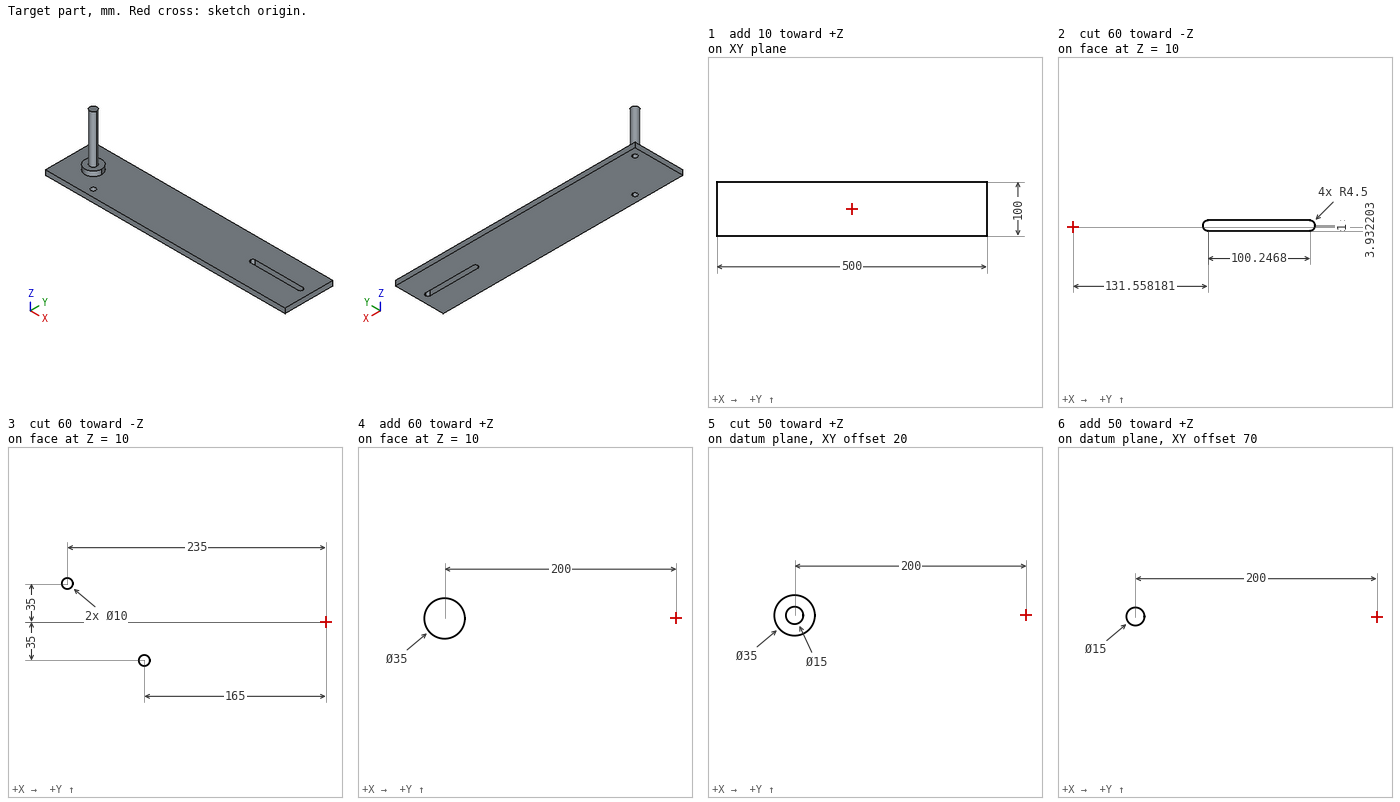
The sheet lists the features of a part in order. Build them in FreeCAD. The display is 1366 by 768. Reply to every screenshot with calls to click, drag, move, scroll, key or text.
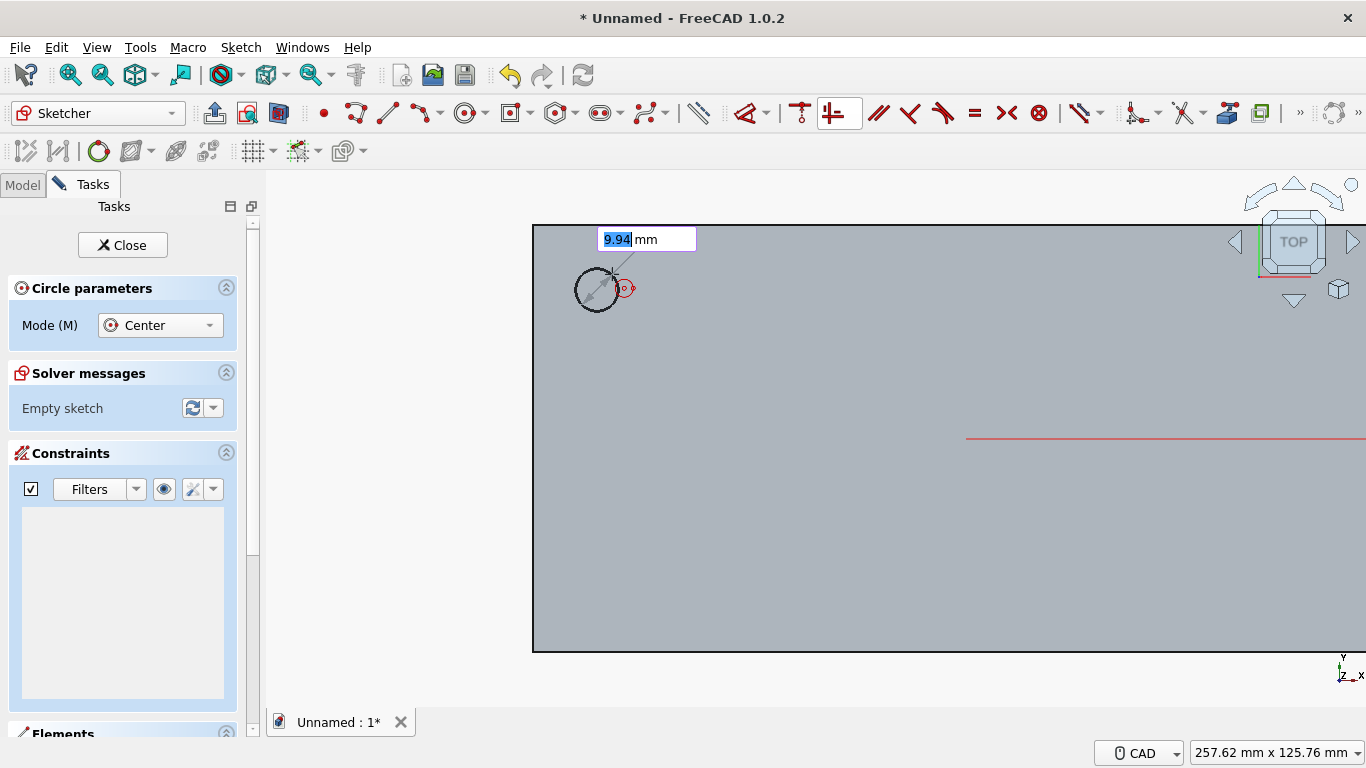
text(10)
key(Return)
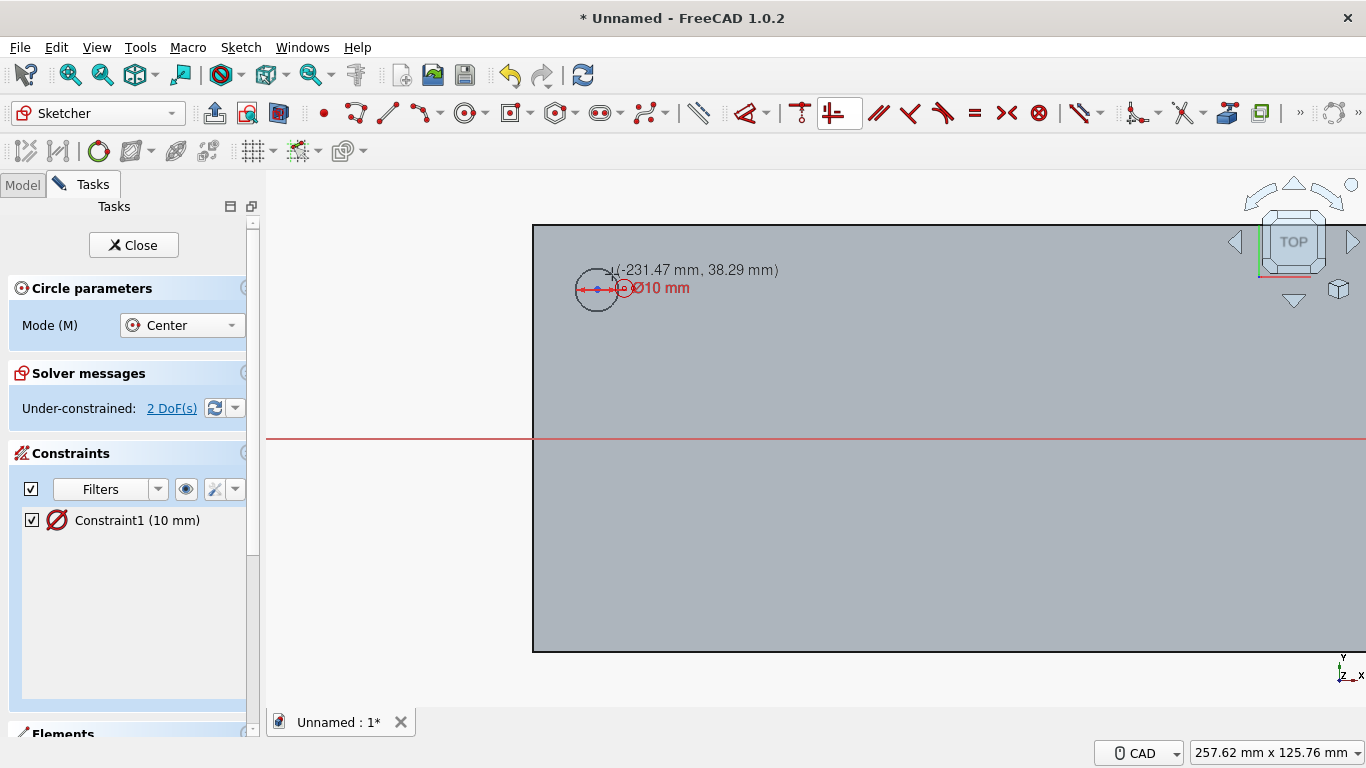
click(896, 588)
move(911, 573)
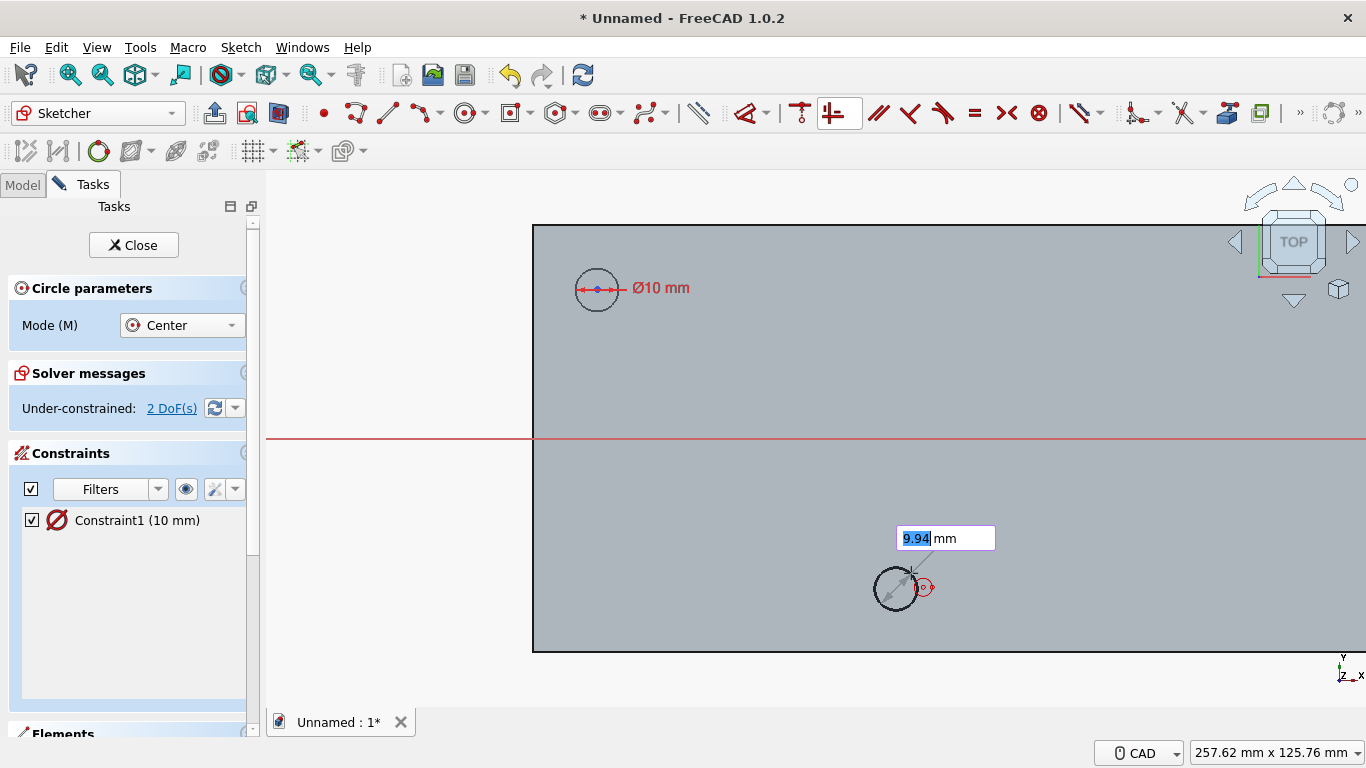
text(10)
key(Return)
key(Escape)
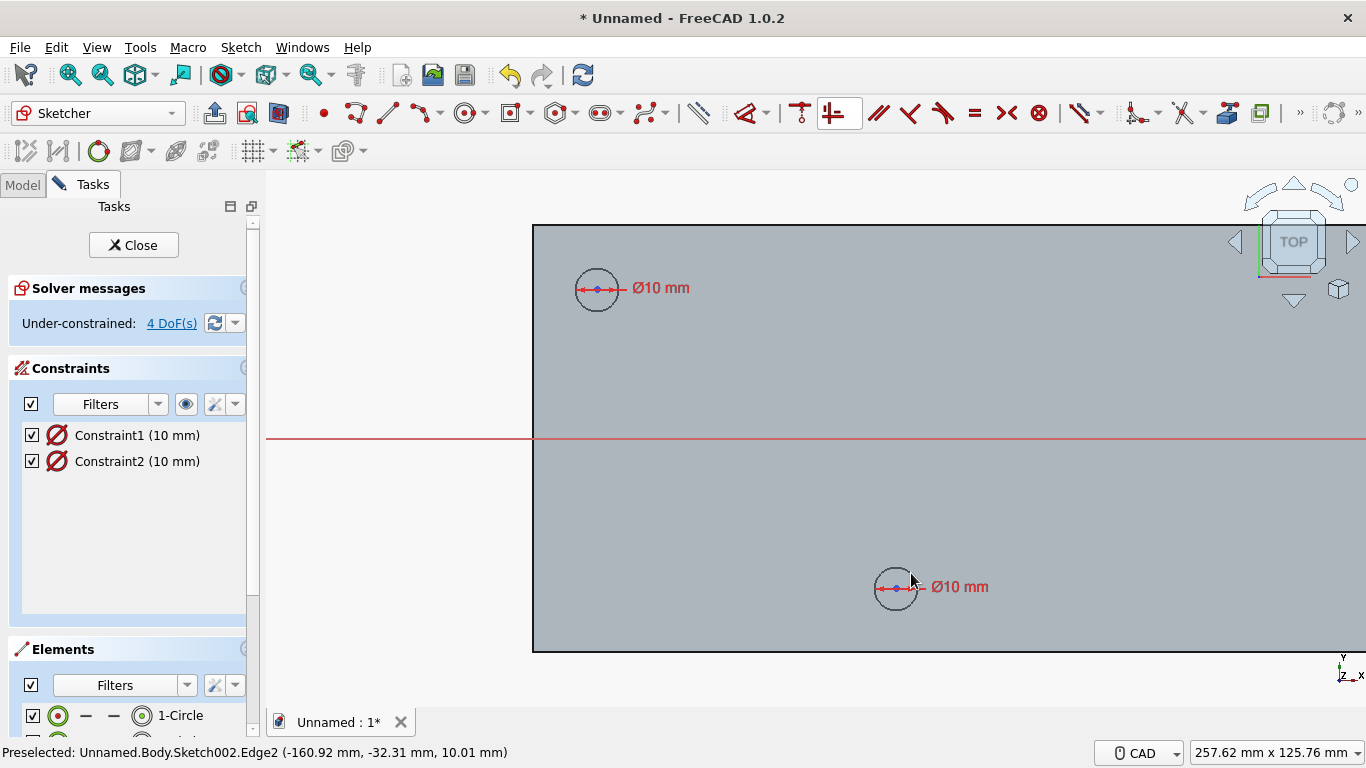
key(d)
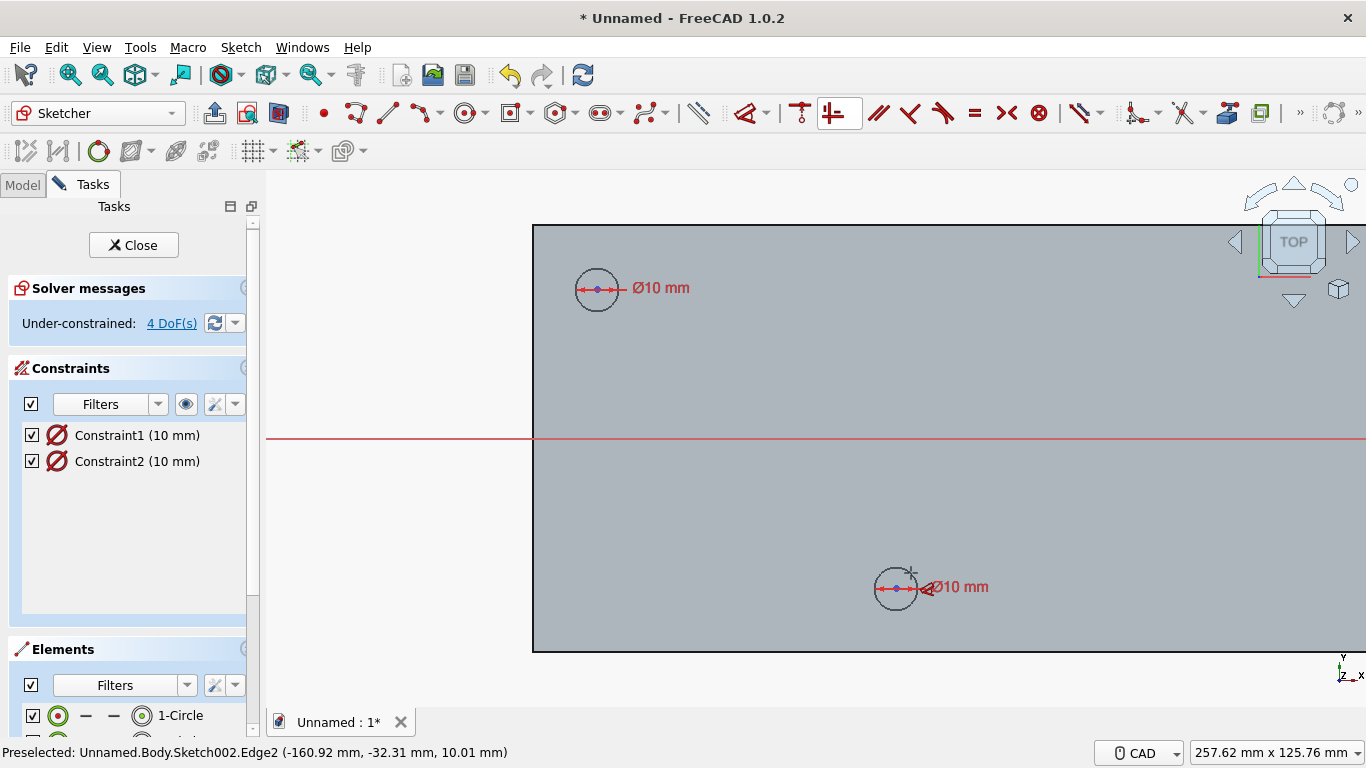
click(597, 290)
click(563, 364)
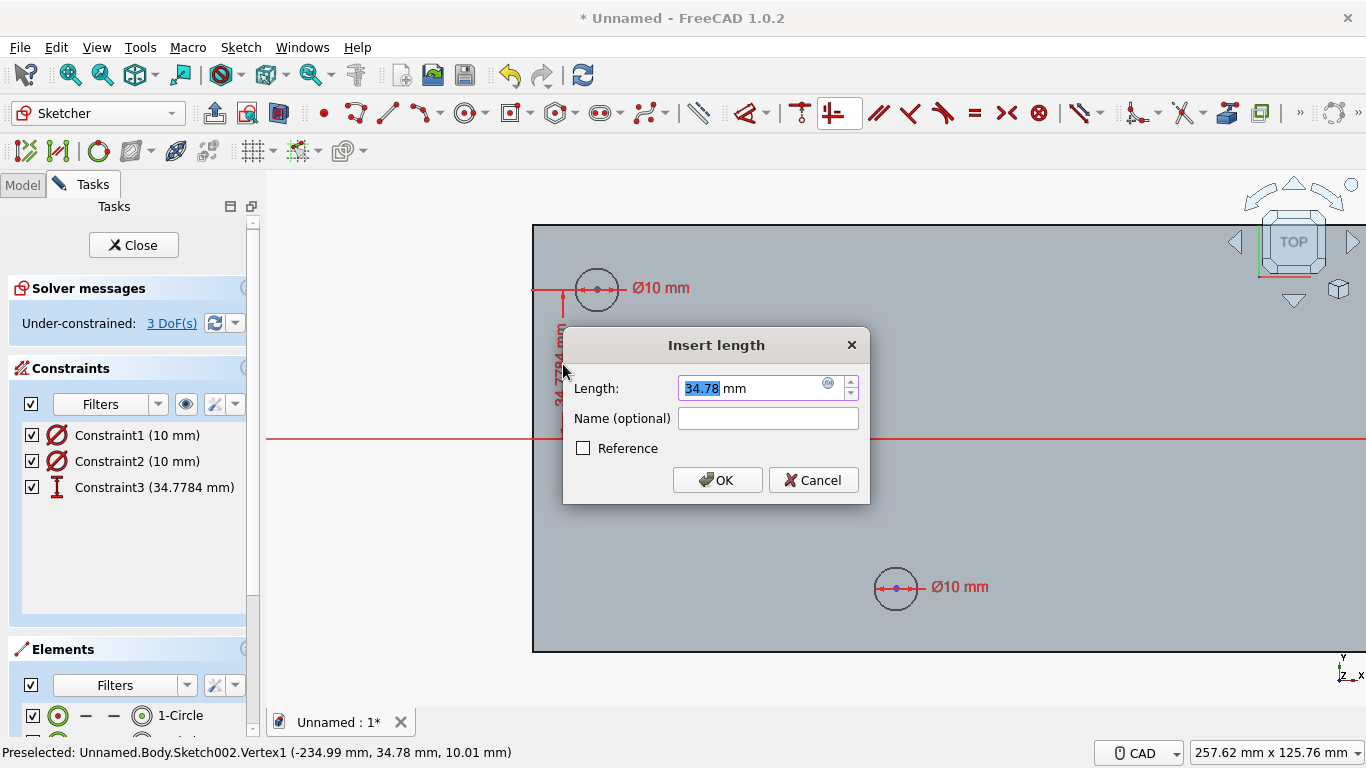
text(35)
key(Return)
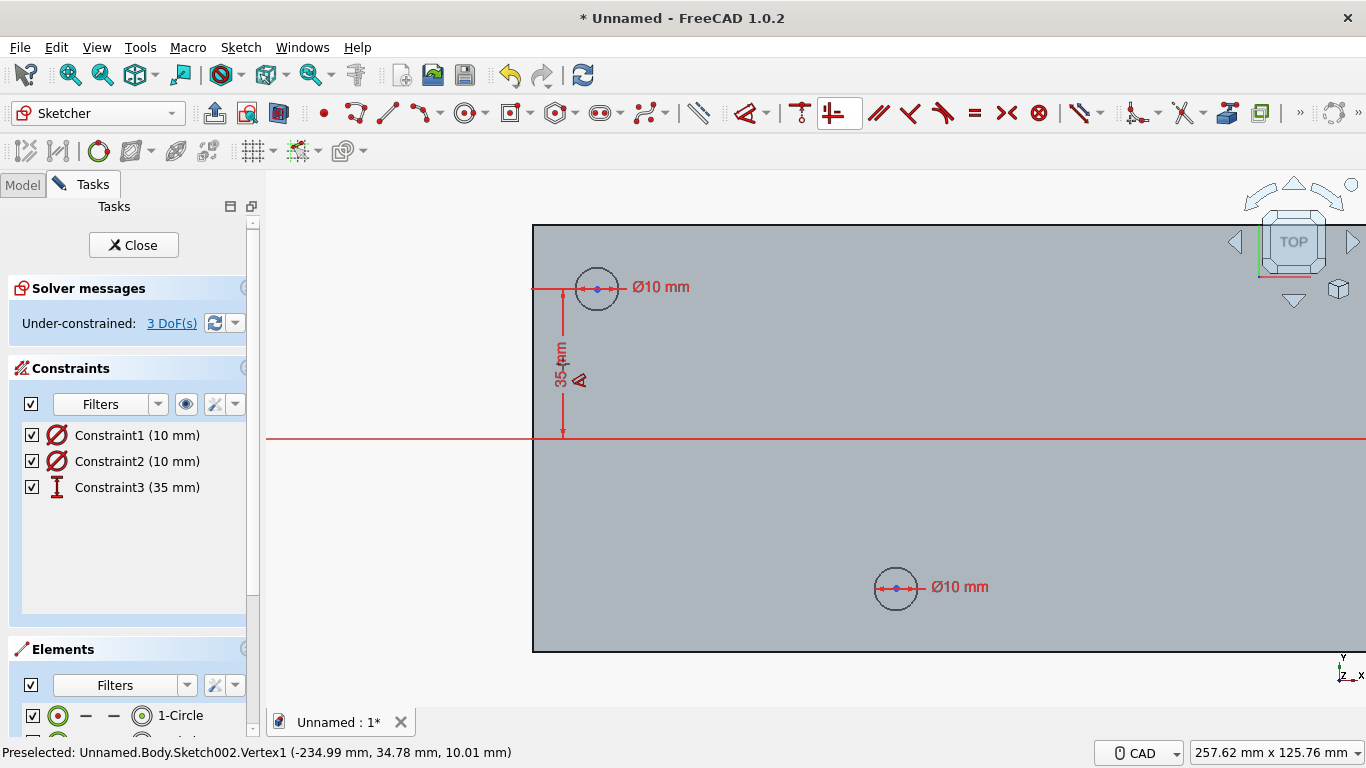
click(896, 589)
click(862, 514)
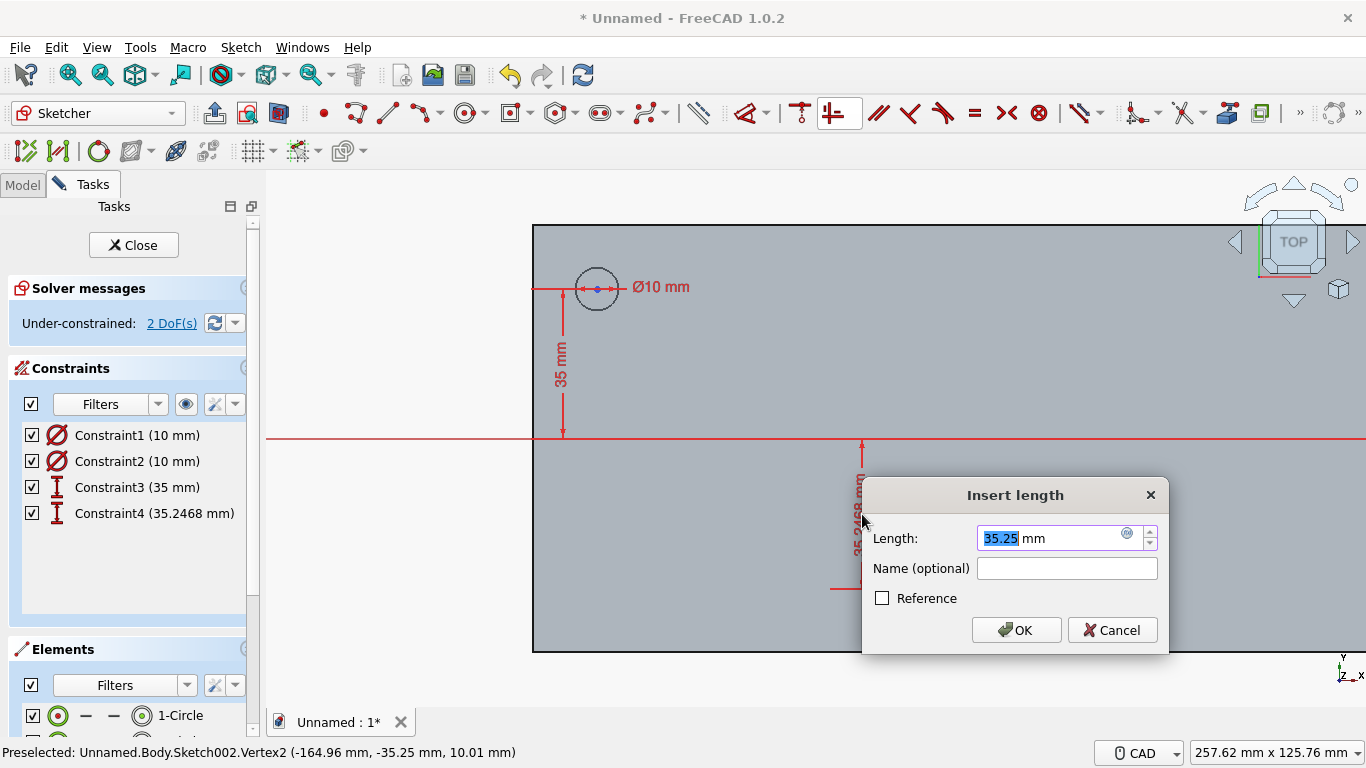
text(35)
key(Return)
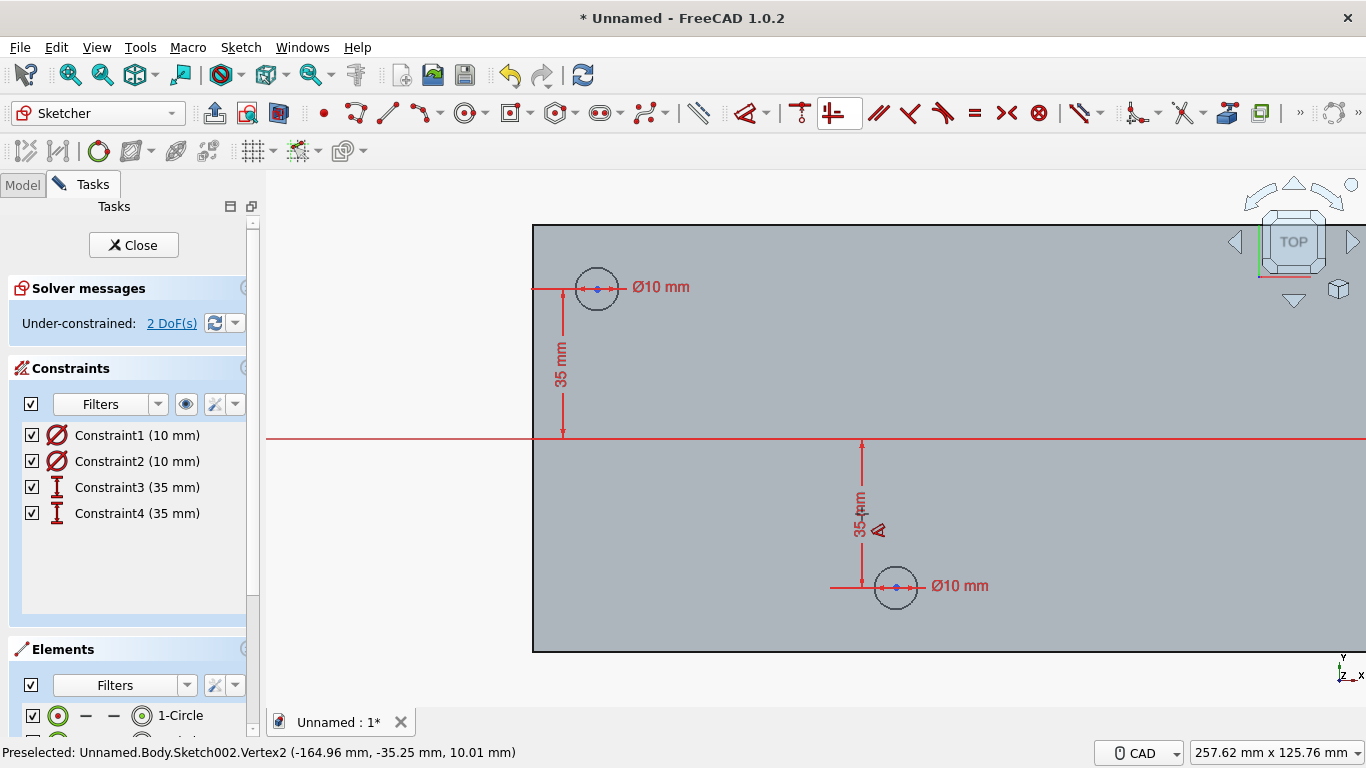
click(597, 289)
click(899, 255)